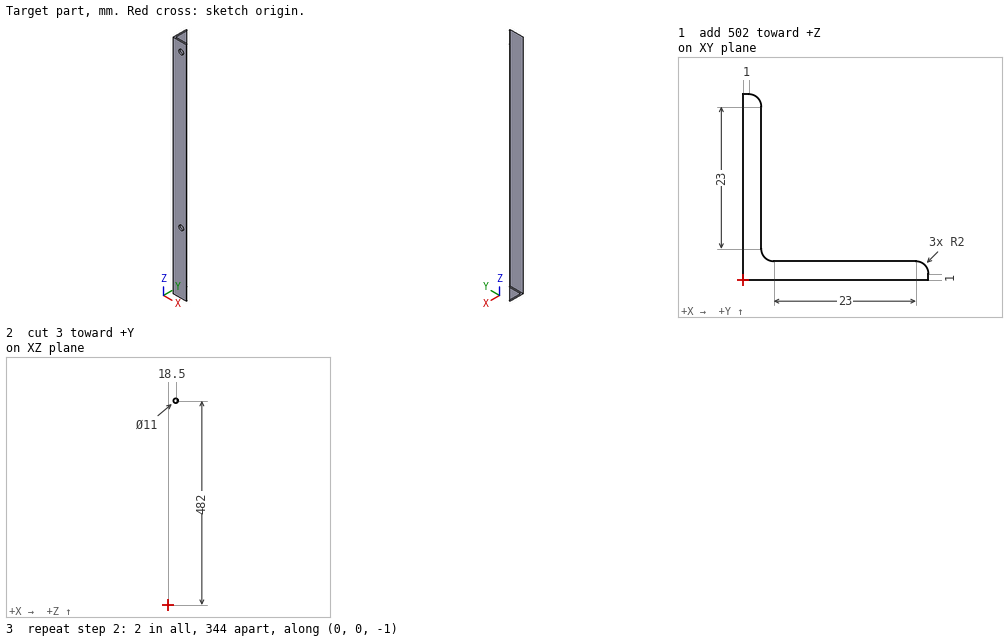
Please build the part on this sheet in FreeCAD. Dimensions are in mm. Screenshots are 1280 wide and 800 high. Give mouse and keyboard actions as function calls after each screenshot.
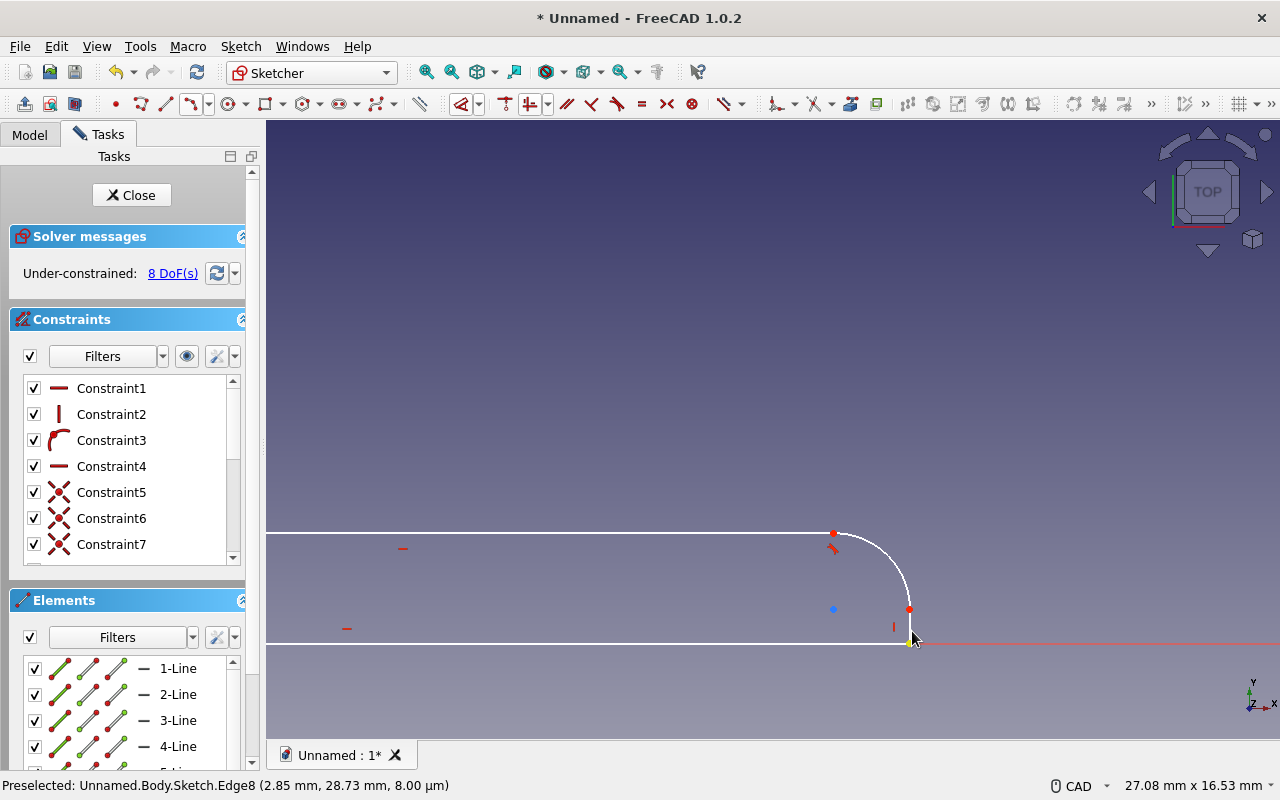
click(910, 630)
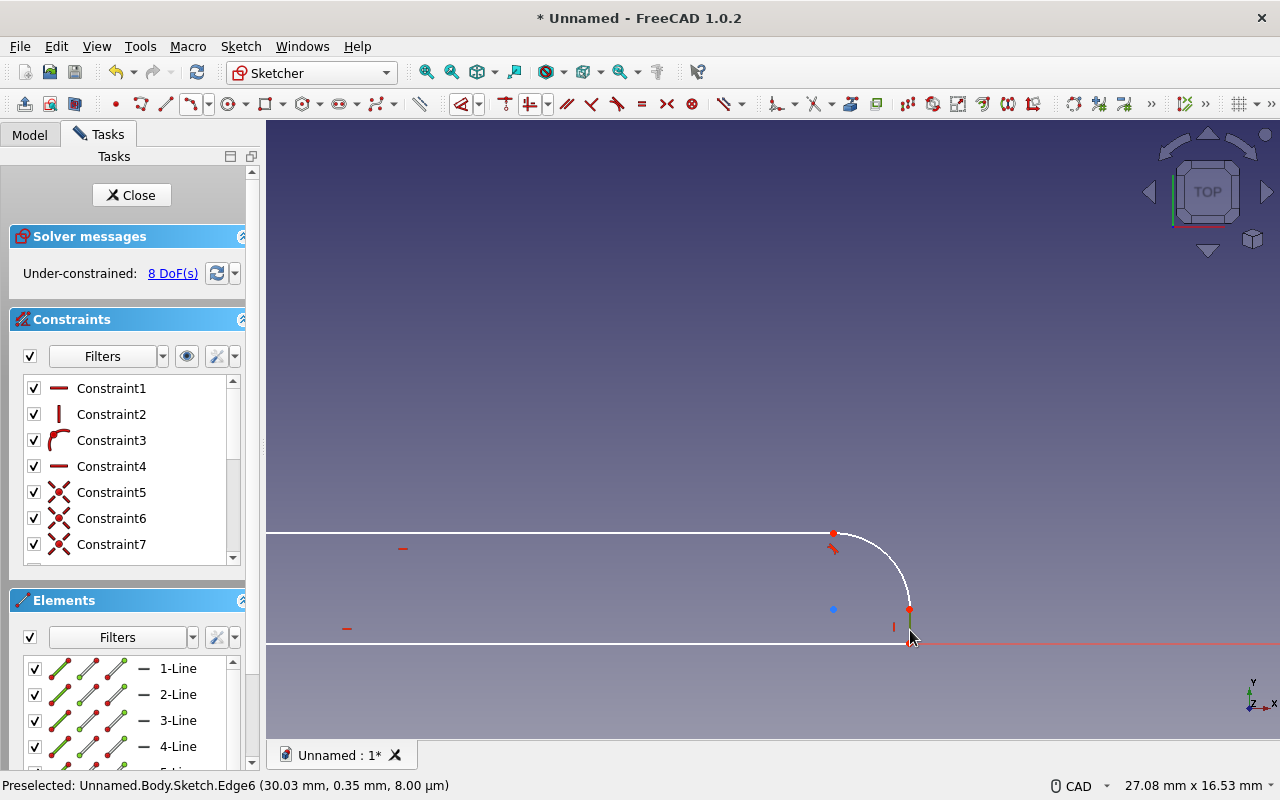
click(902, 575)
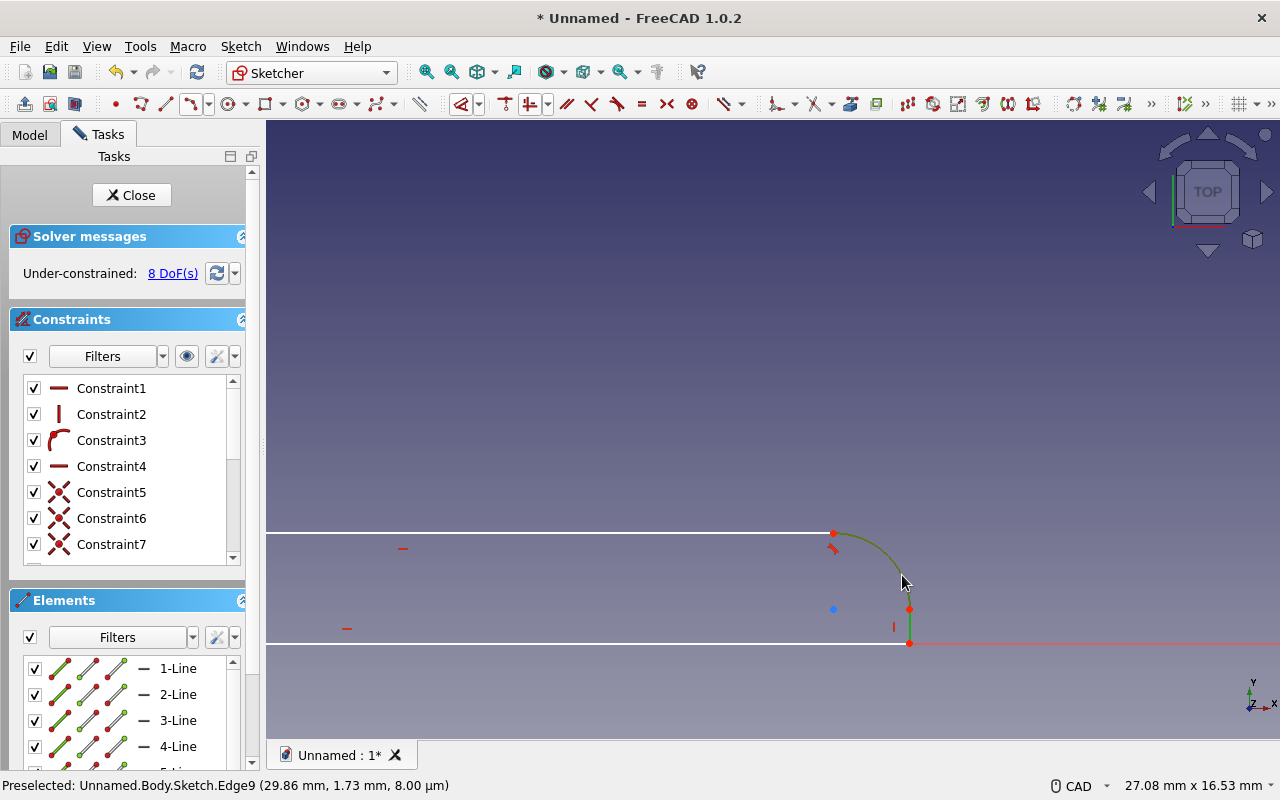
click(617, 104)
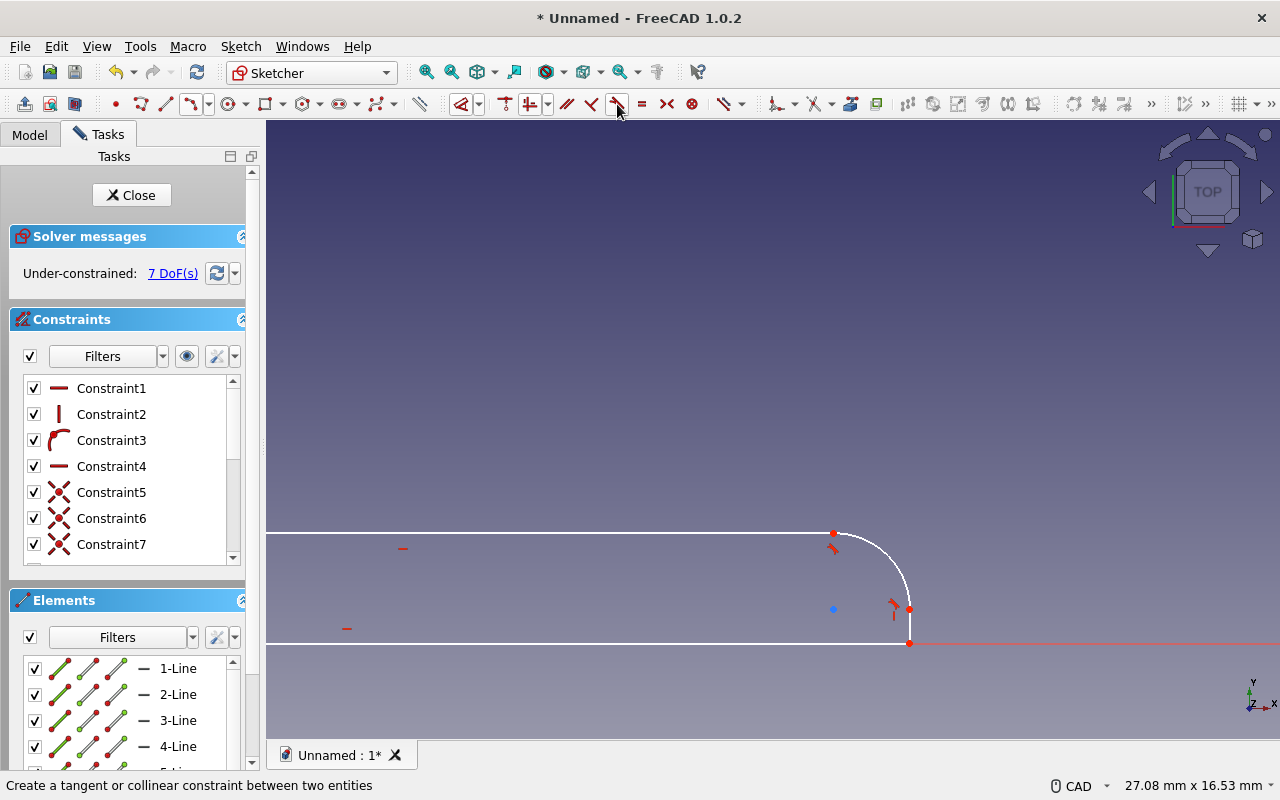
scroll(912, 632, down, 5)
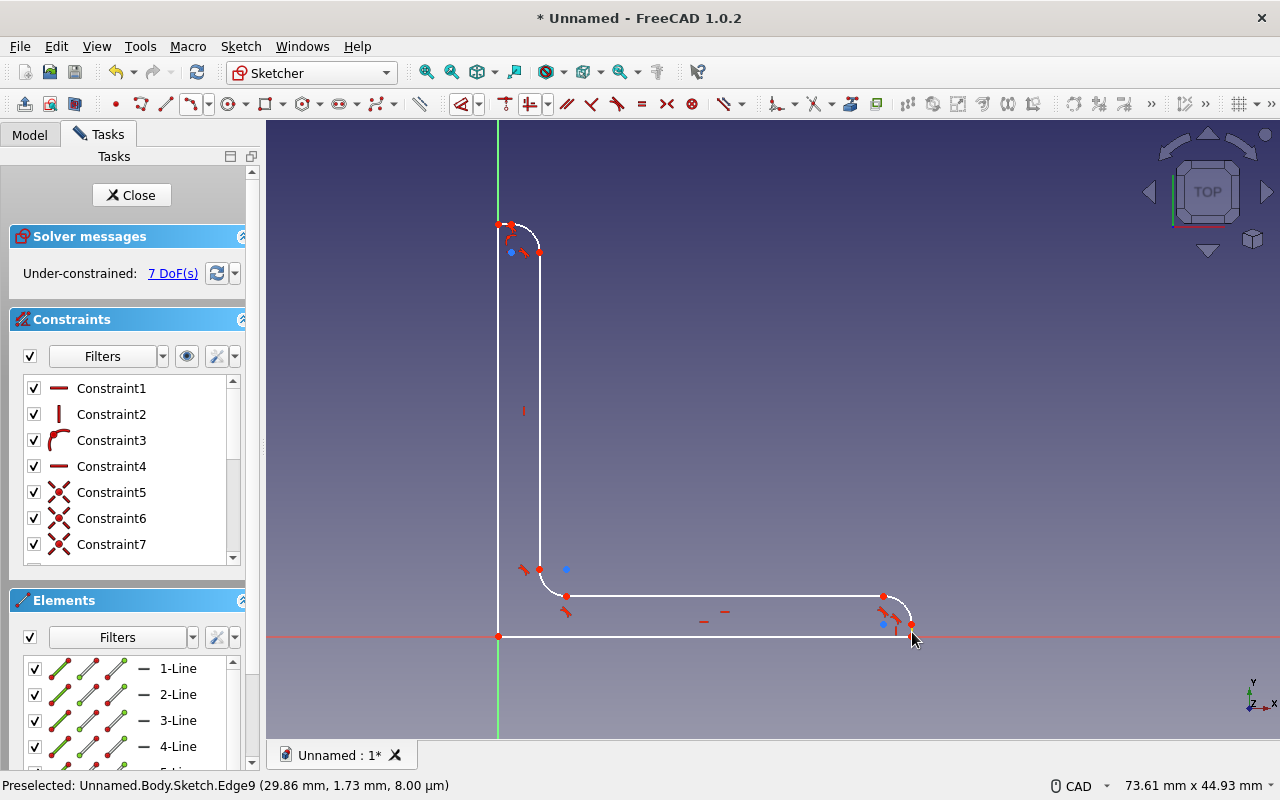
click(543, 581)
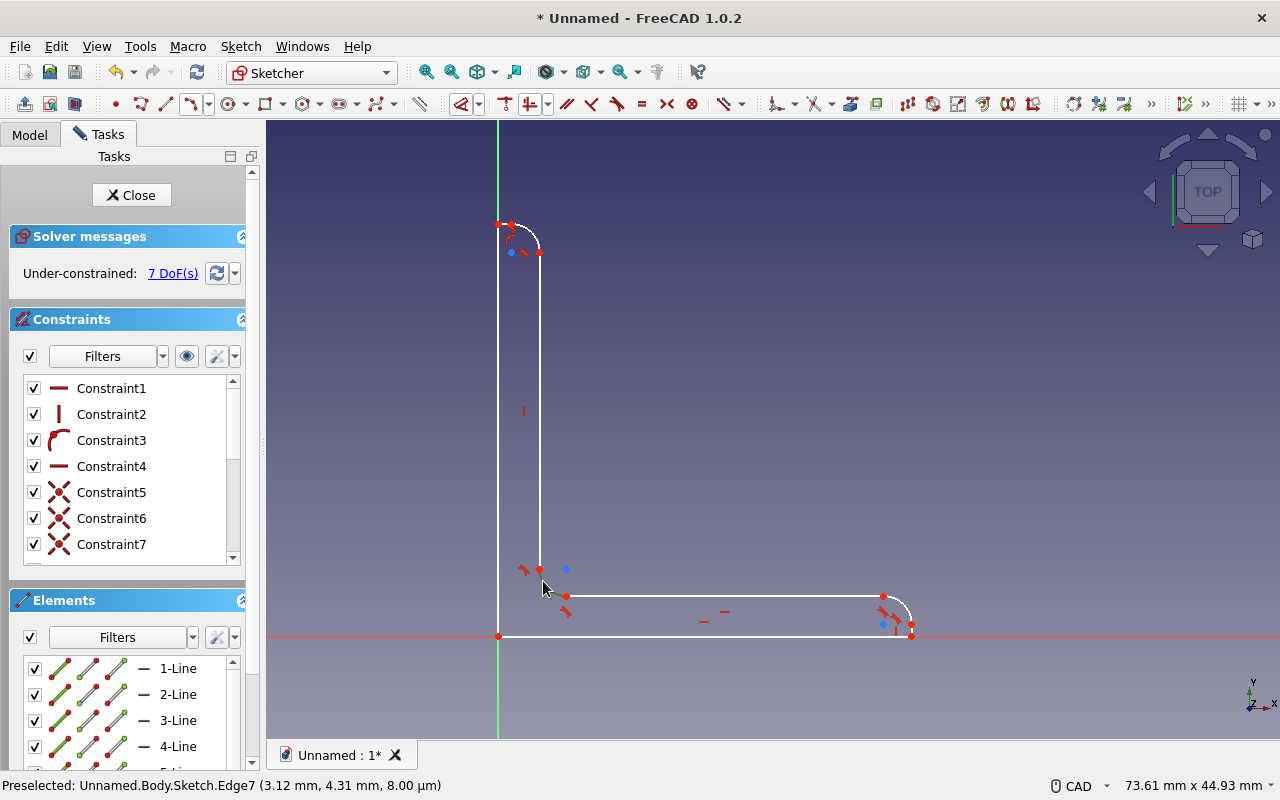
click(537, 239)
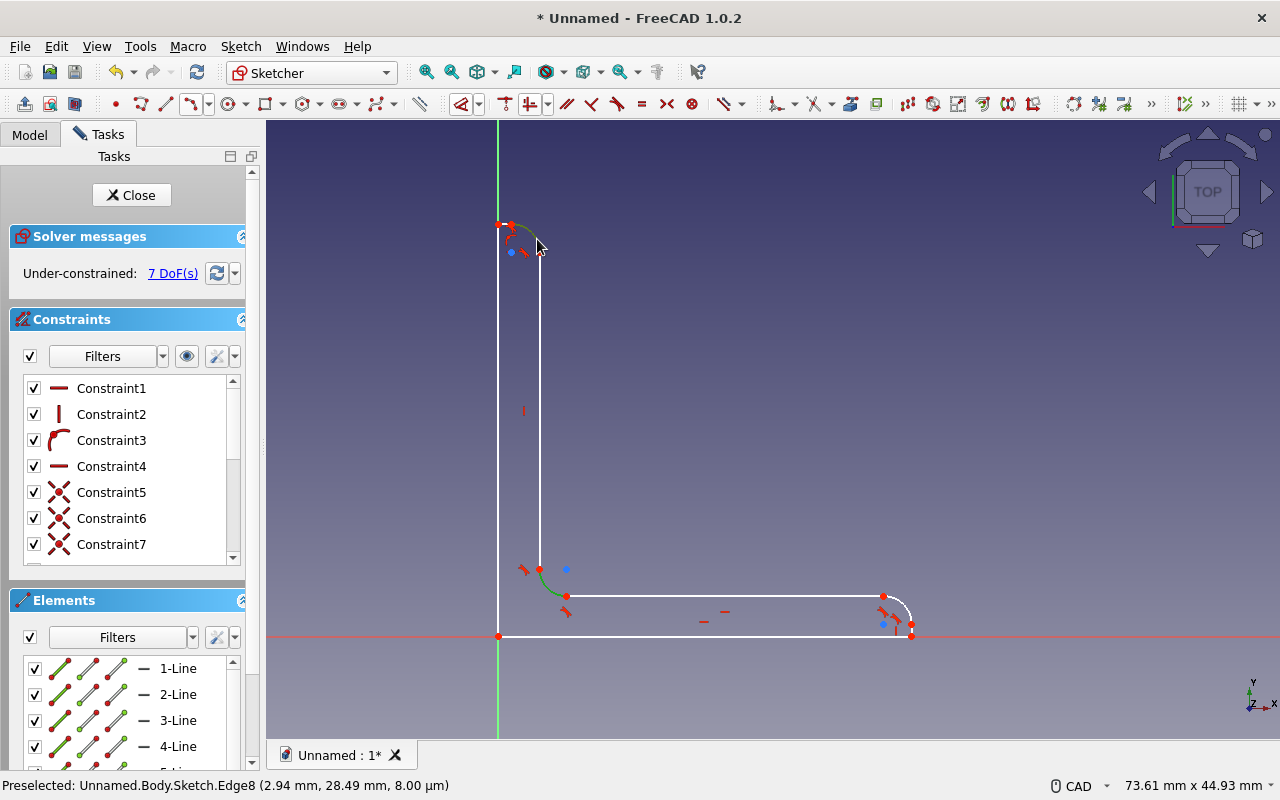
click(909, 611)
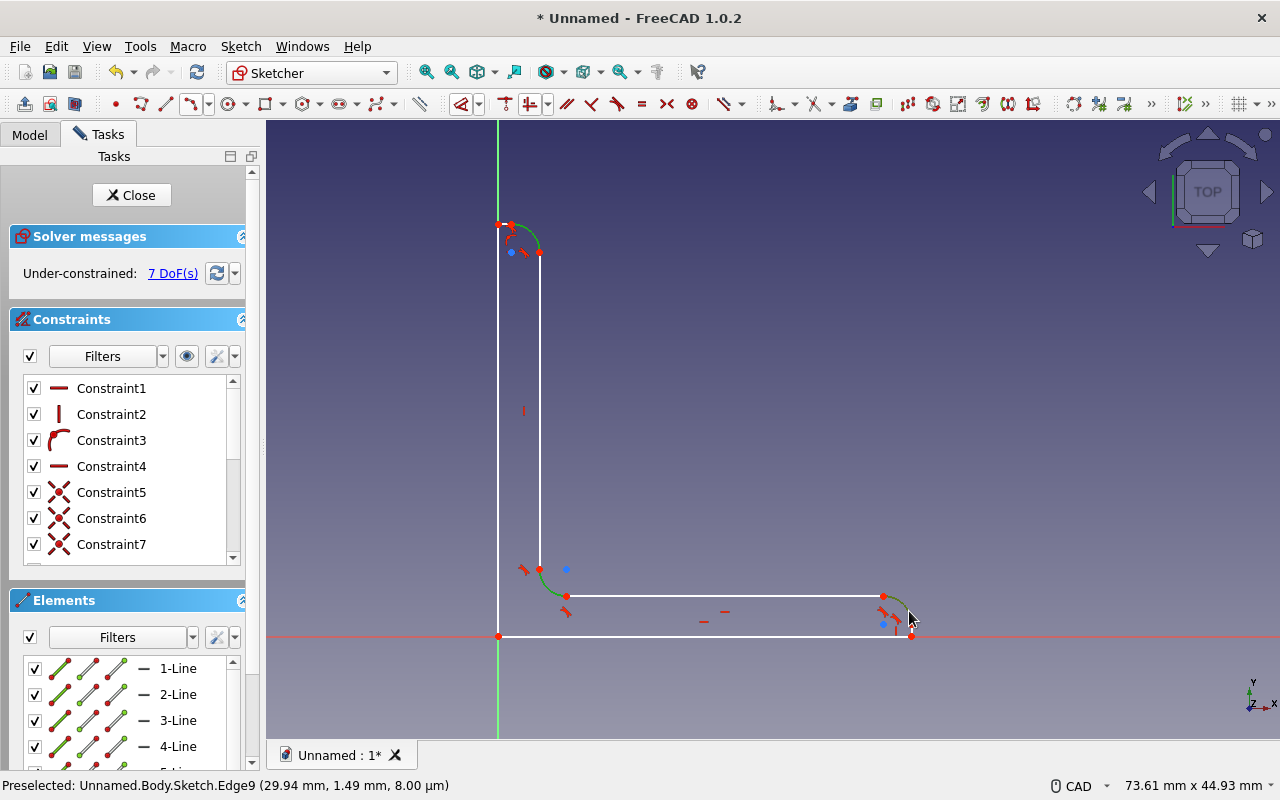
click(642, 104)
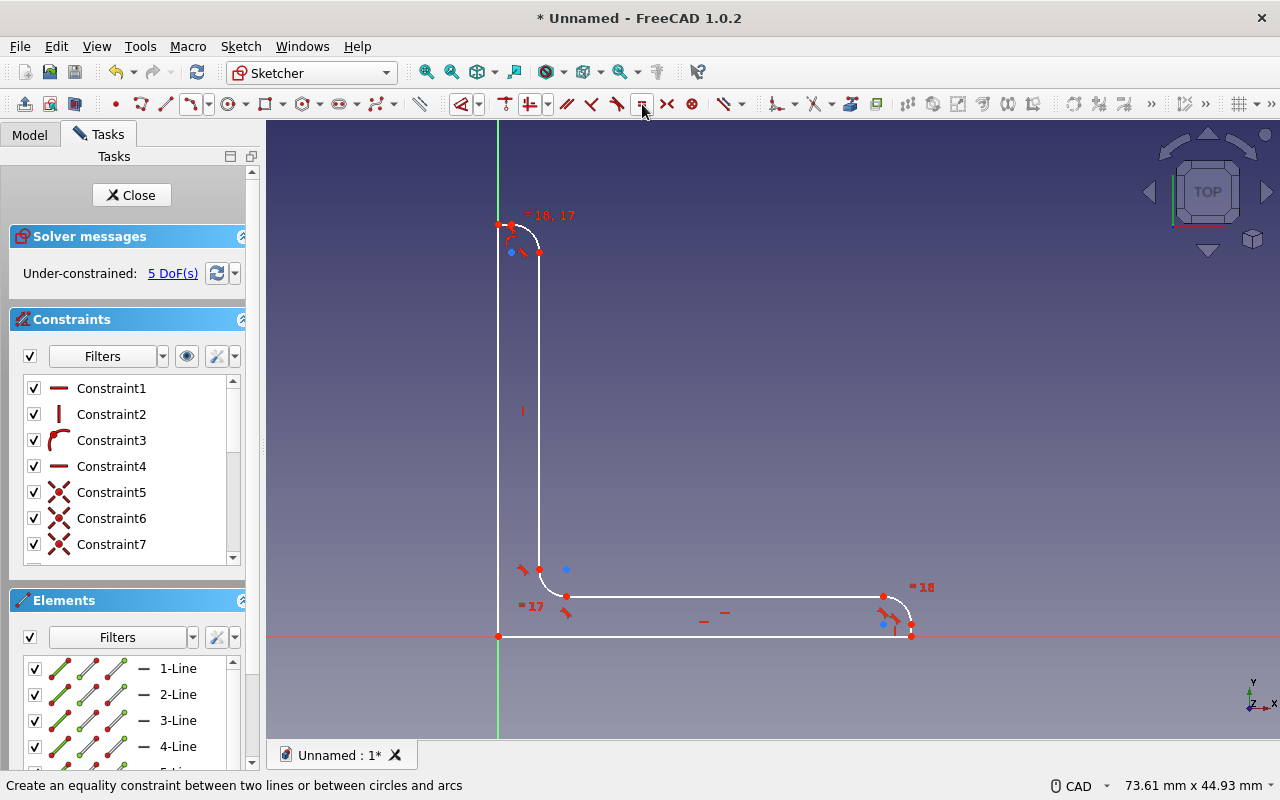
scroll(542, 582, up, 2)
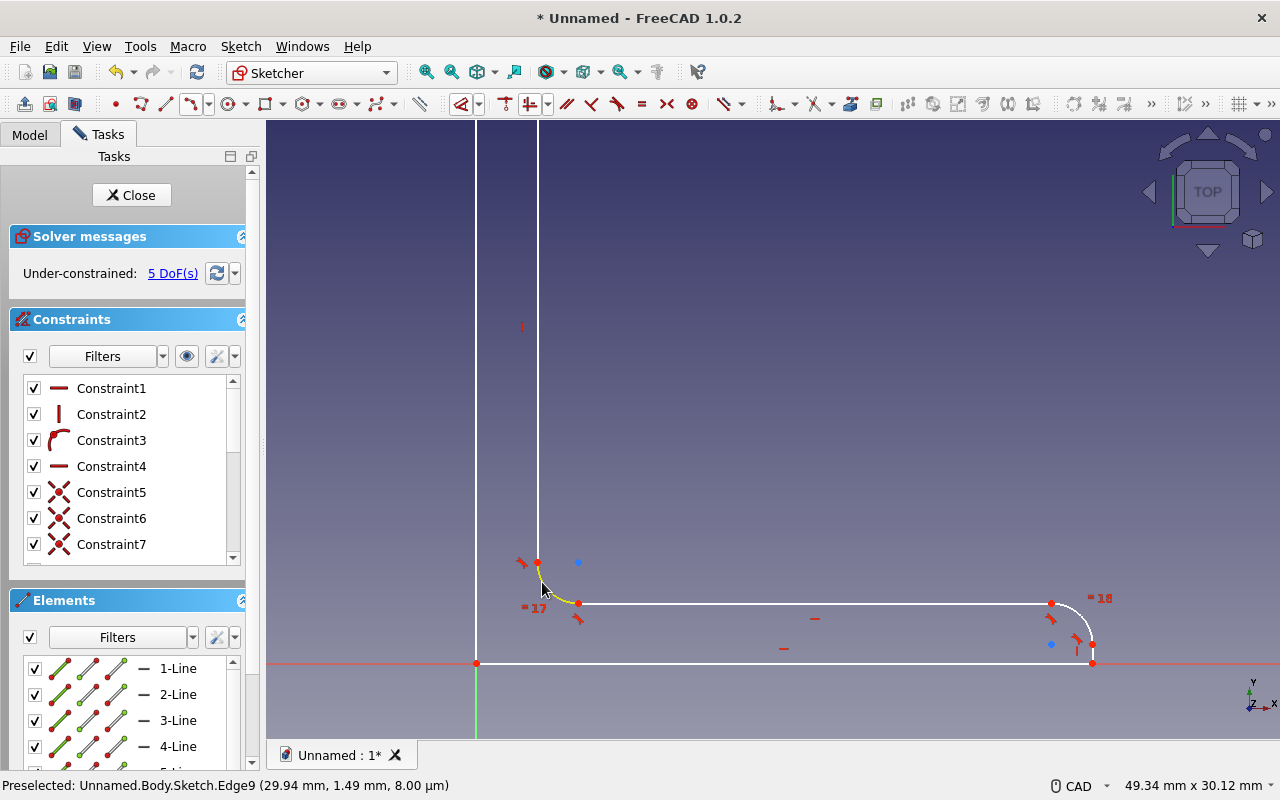
click(542, 581)